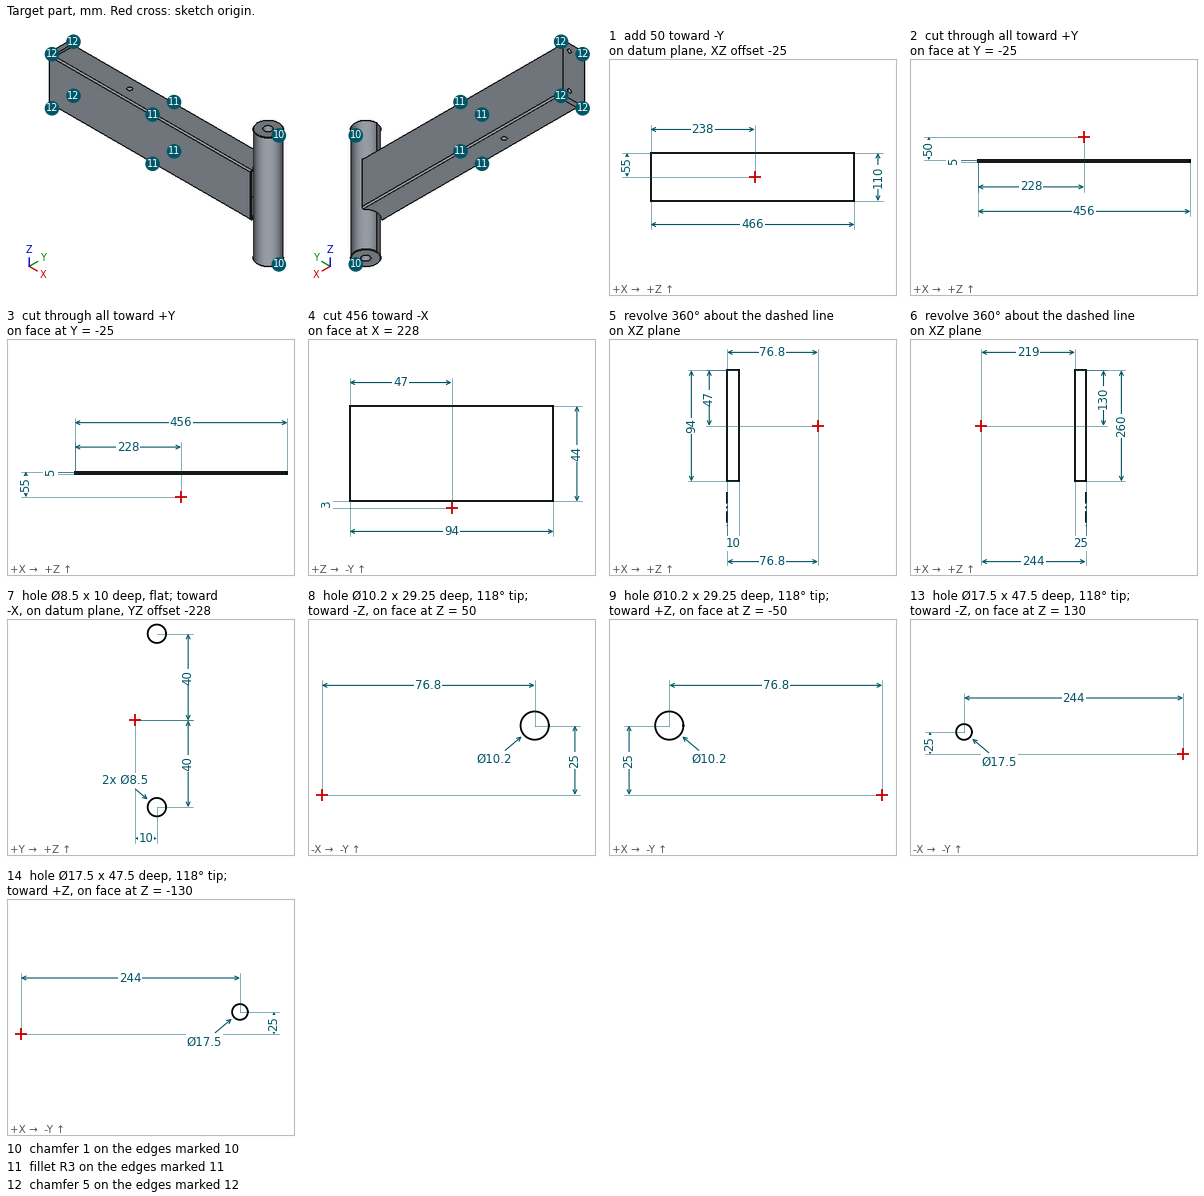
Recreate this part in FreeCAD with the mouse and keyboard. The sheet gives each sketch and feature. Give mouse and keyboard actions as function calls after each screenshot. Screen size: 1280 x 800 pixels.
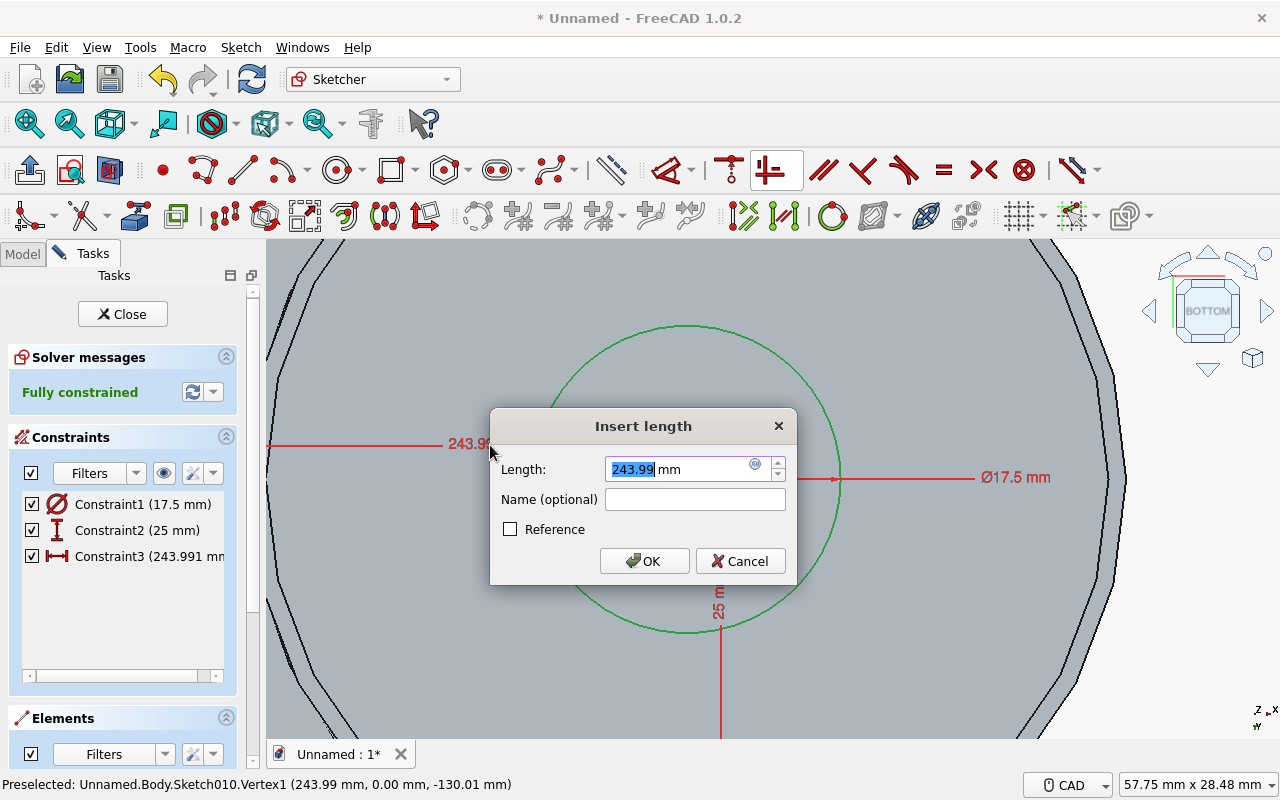
text(244)
key(Return)
key(Escape)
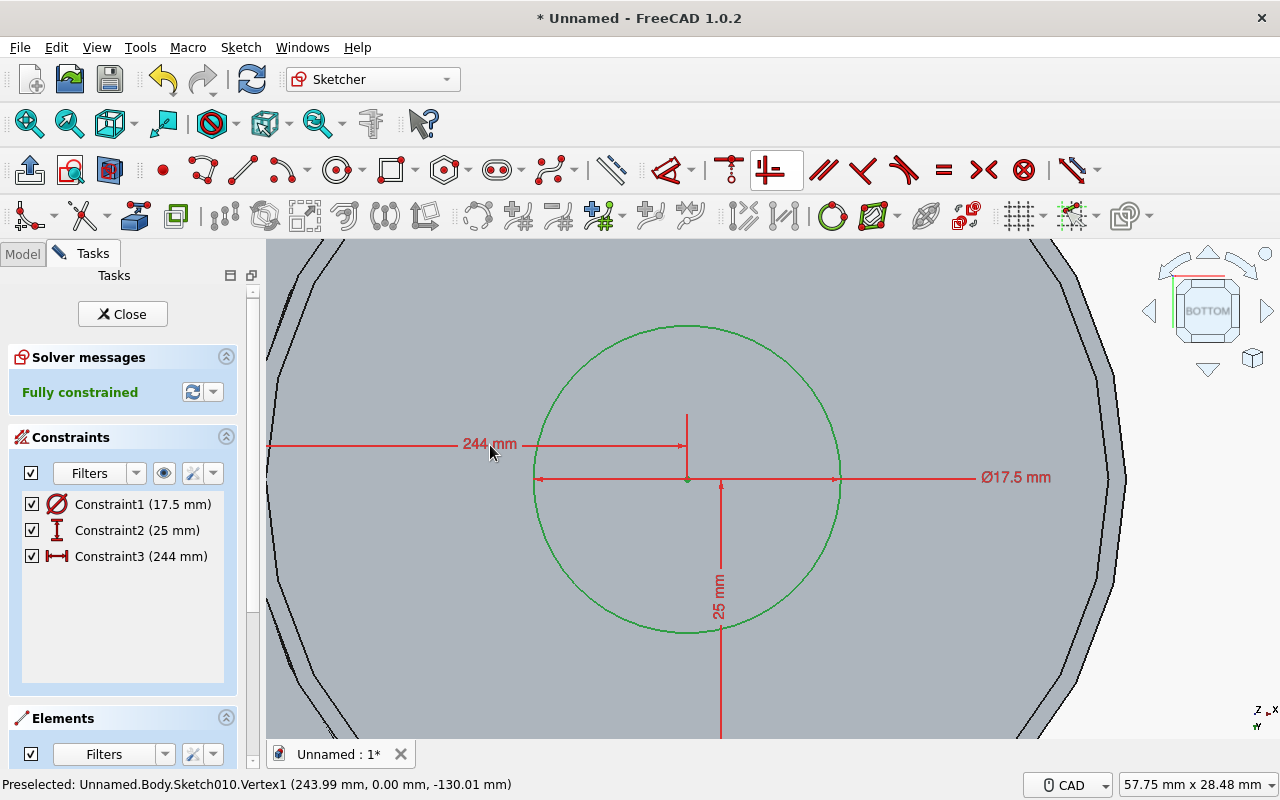
click(123, 314)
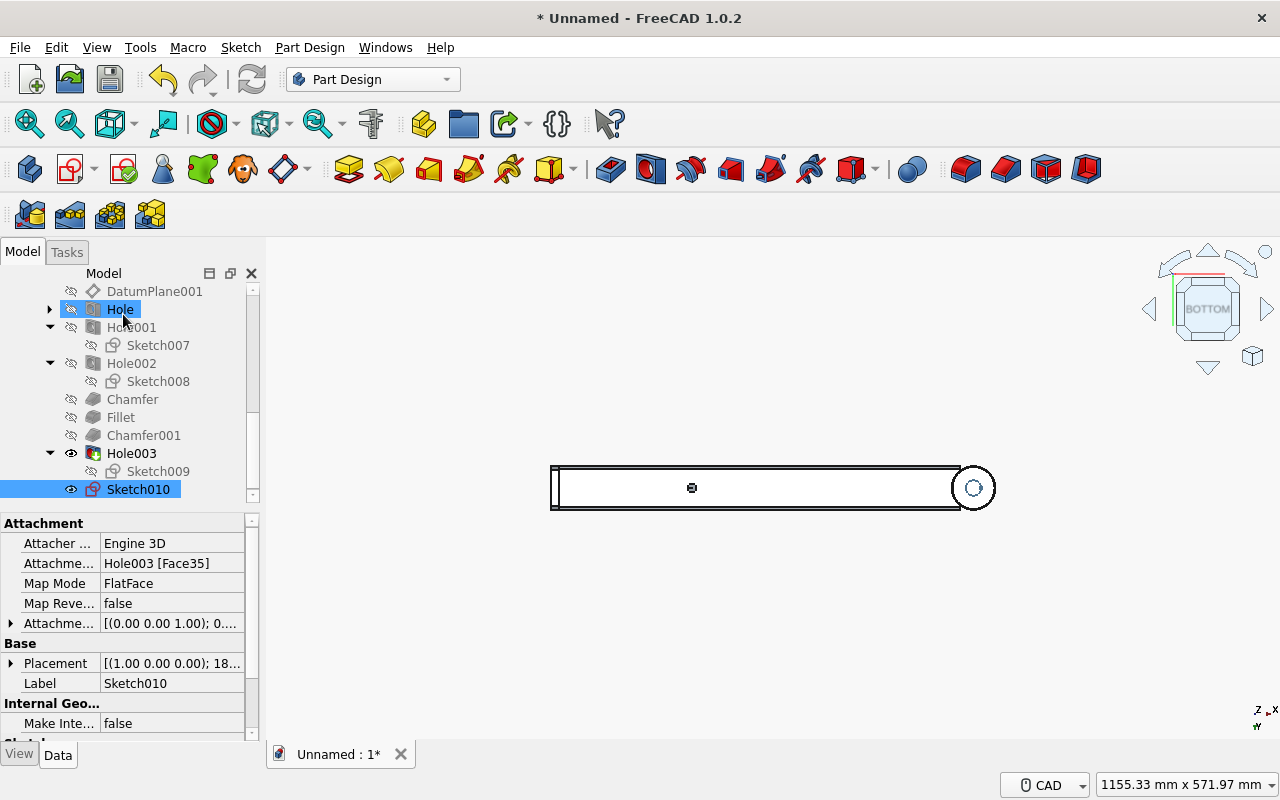
click(652, 170)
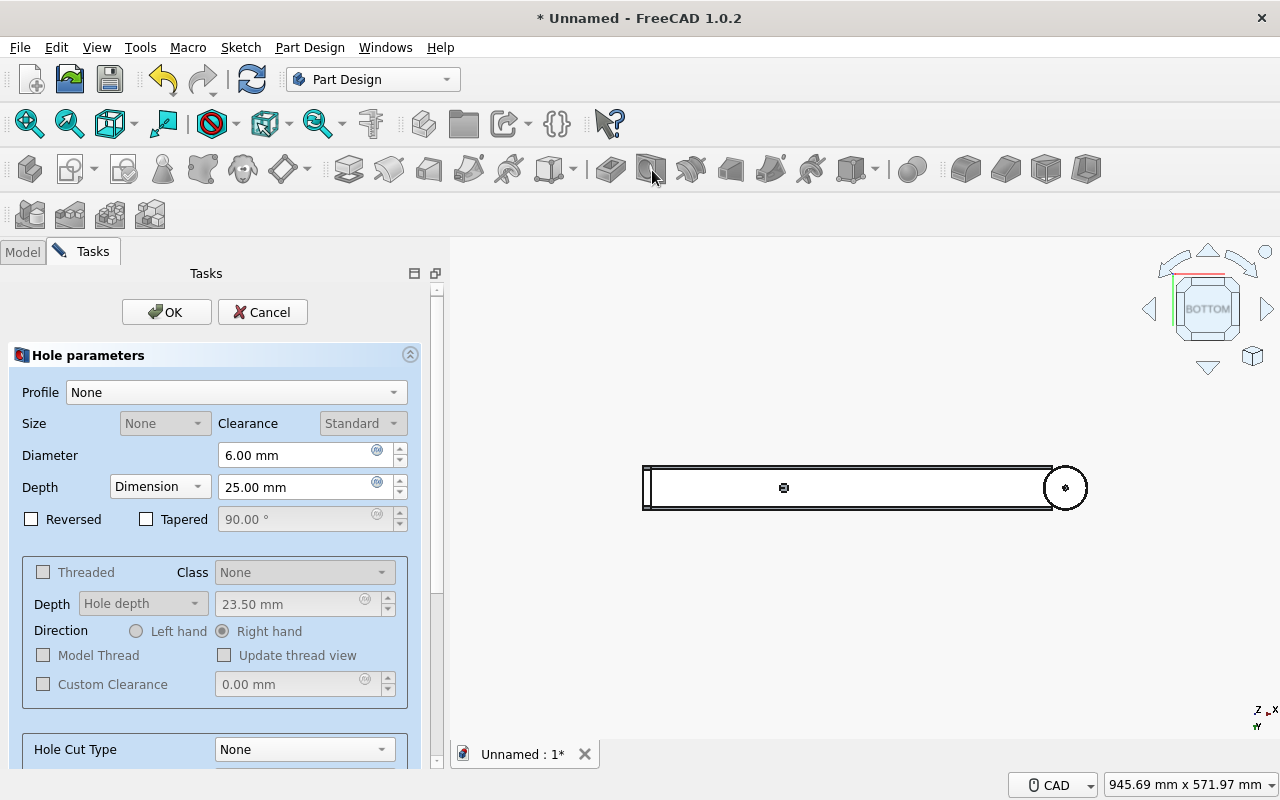
triple_click(305, 455)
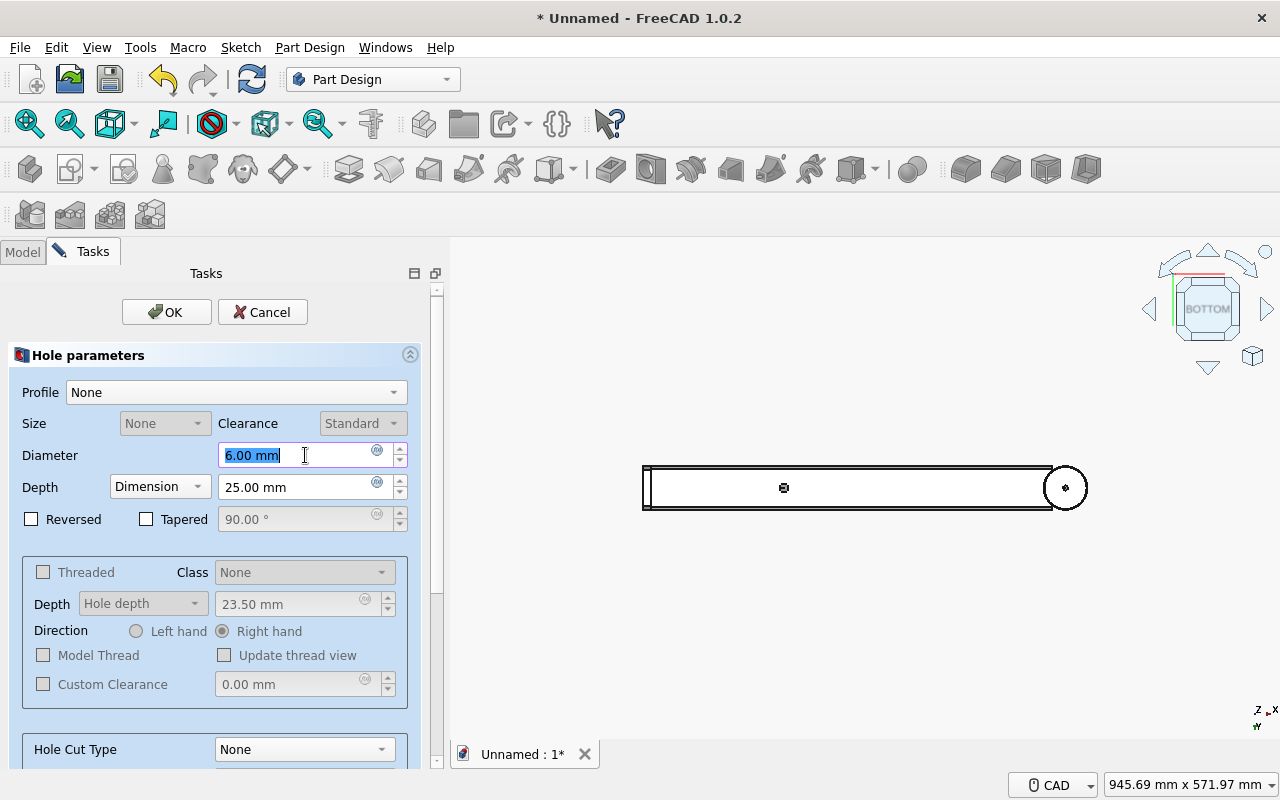
text(17.5)
key(Tab)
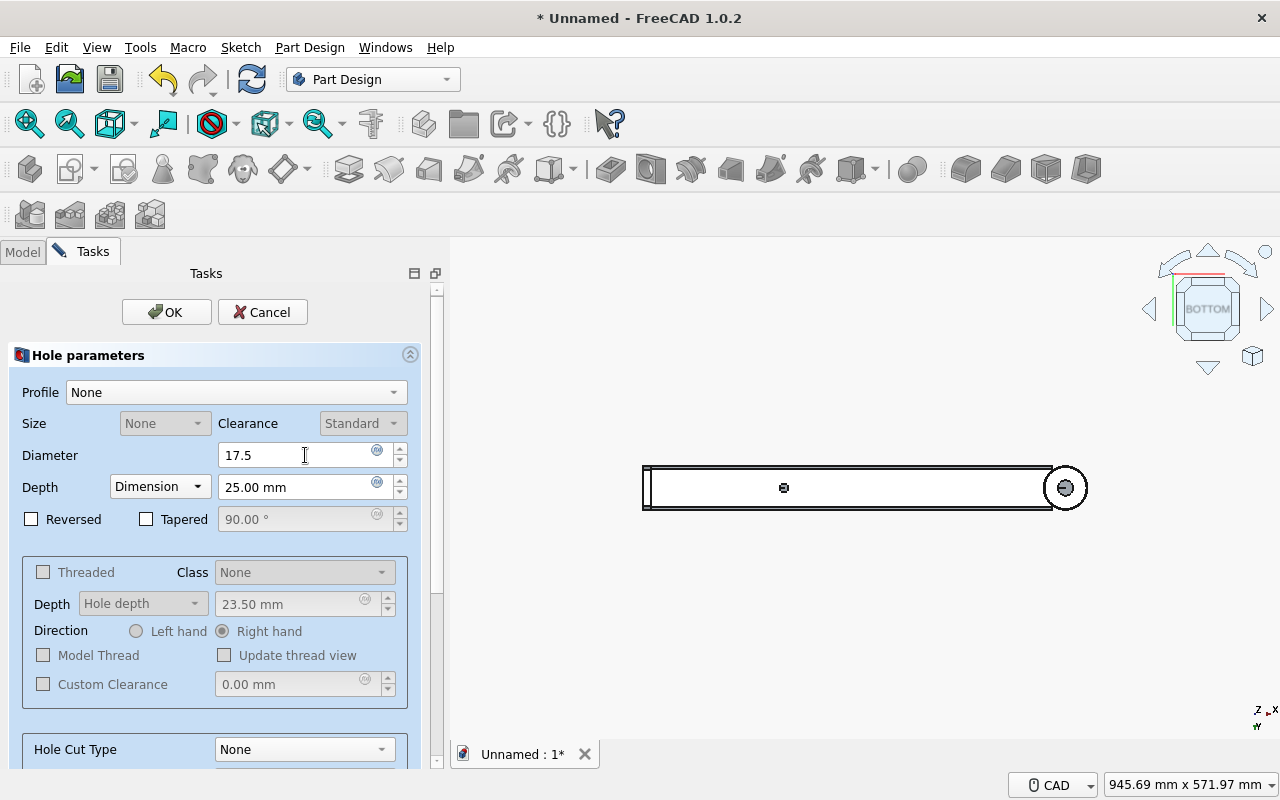
triple_click(305, 487)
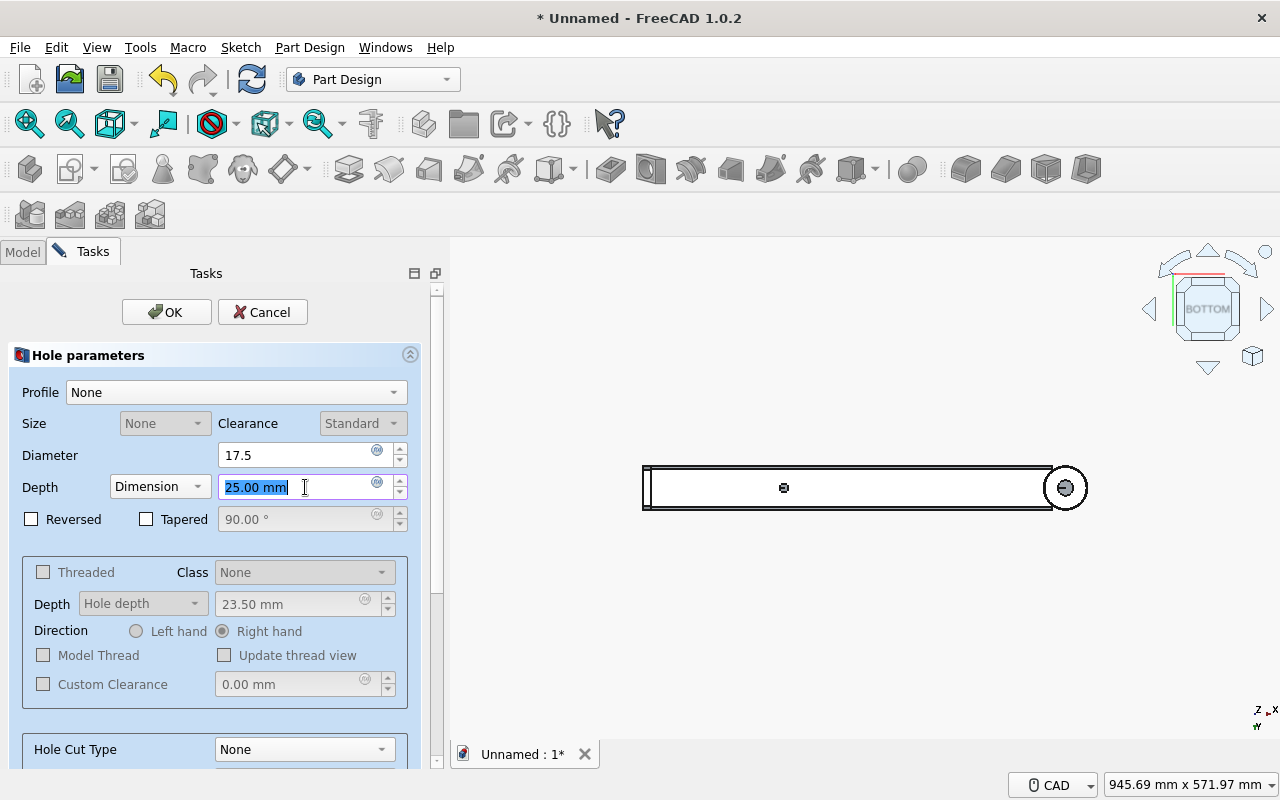
text(47.5)
key(Tab)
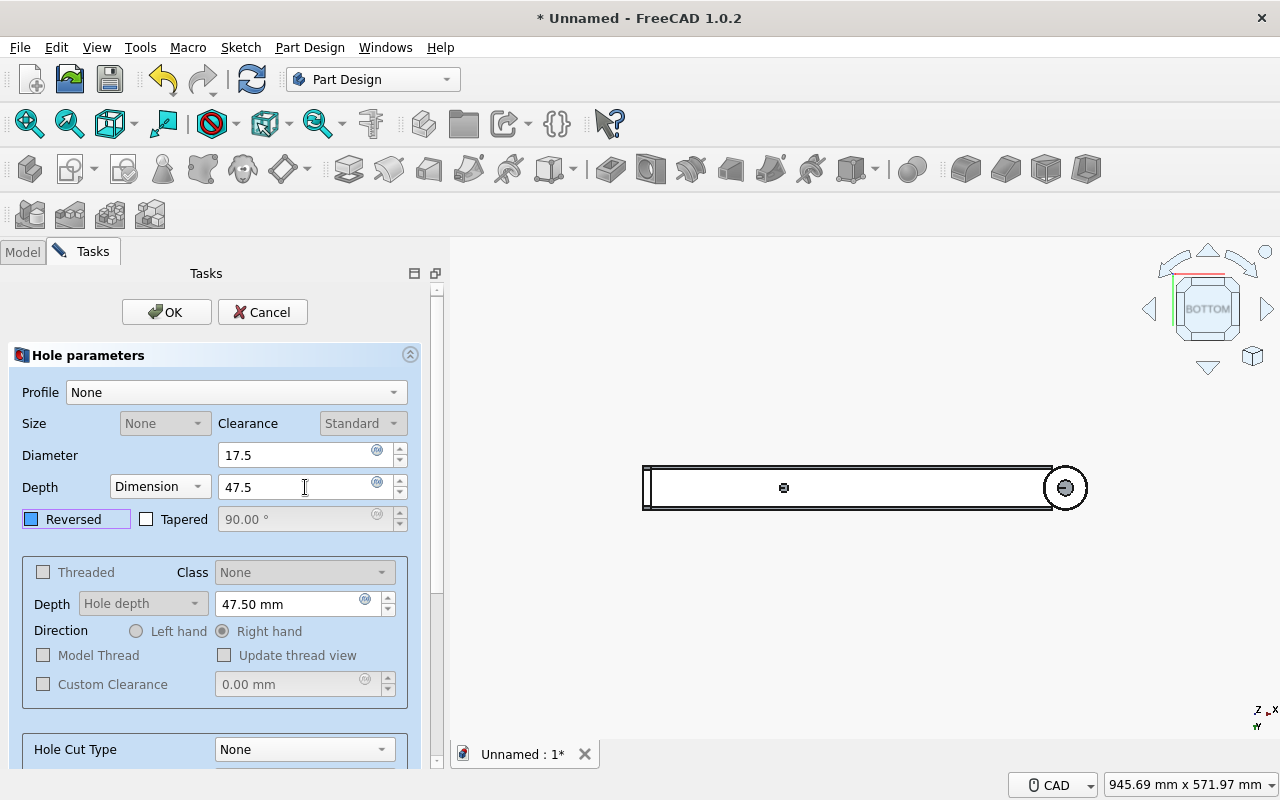
click(167, 312)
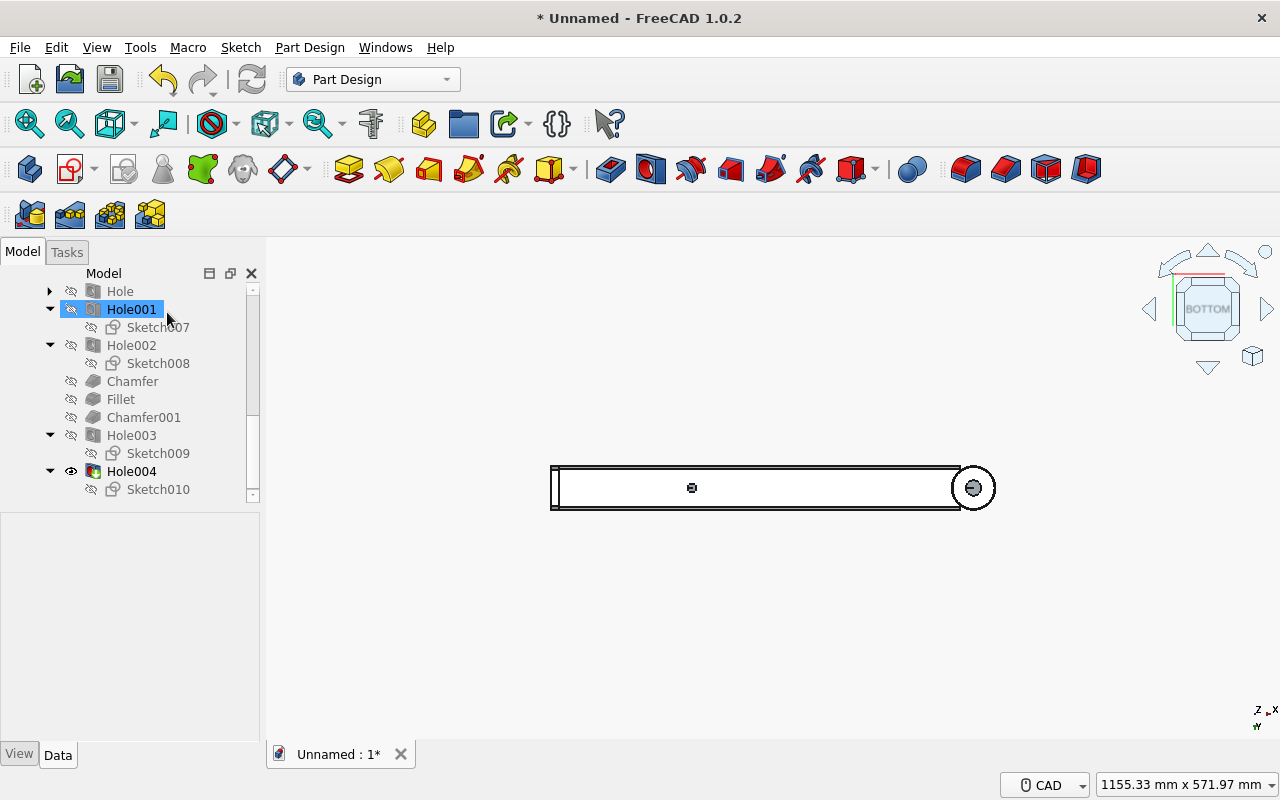
key(0)